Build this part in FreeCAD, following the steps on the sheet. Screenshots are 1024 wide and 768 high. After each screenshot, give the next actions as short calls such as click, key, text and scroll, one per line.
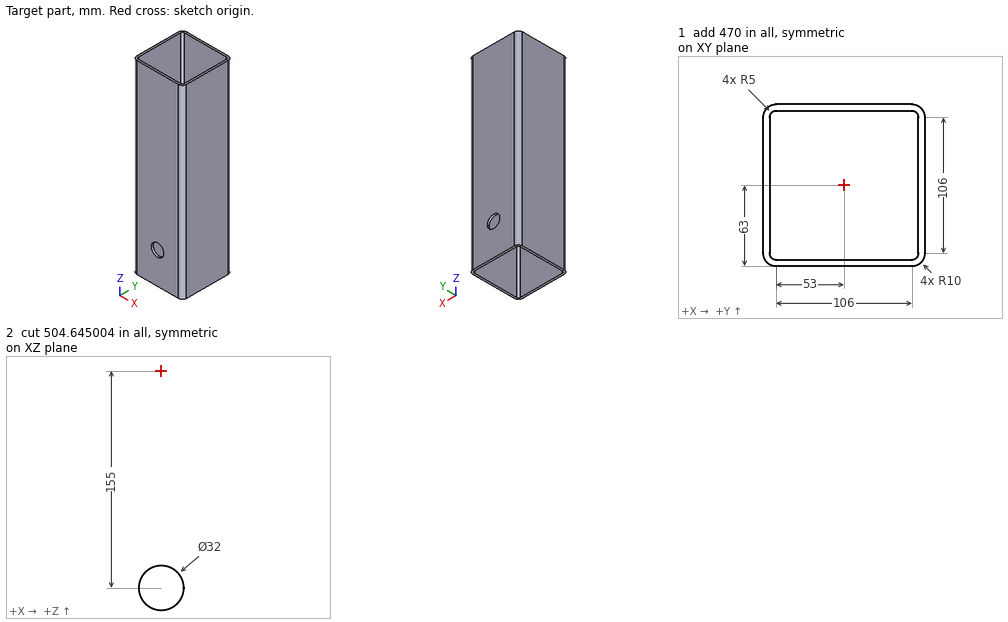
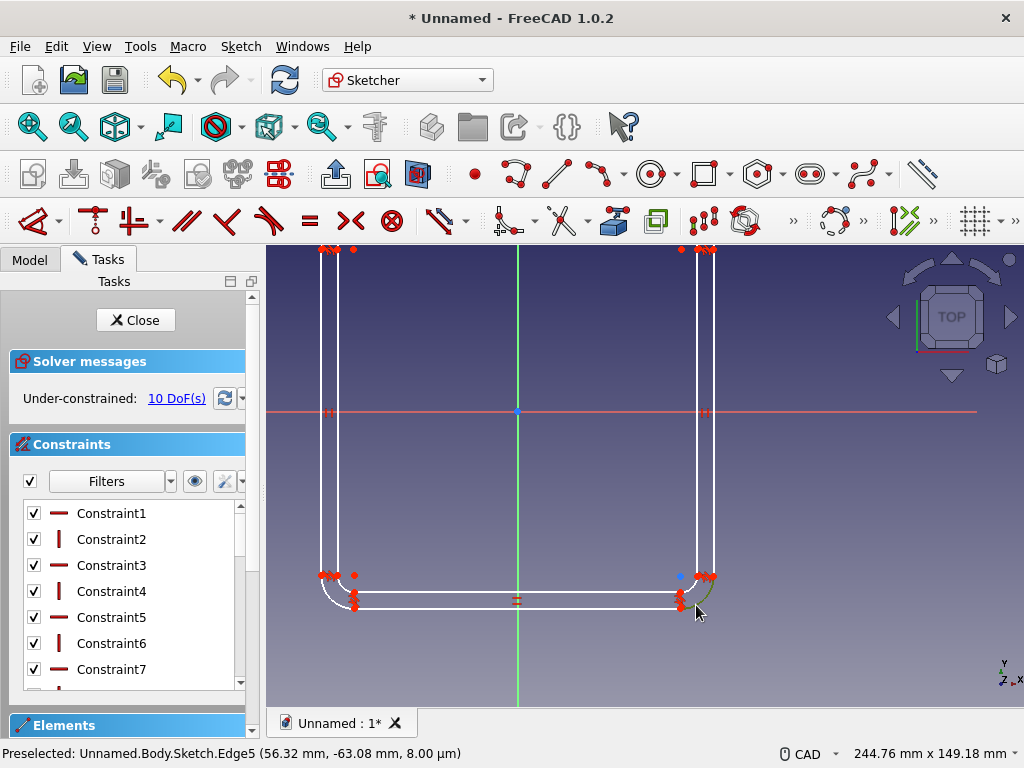
scroll(696, 607, down, 2)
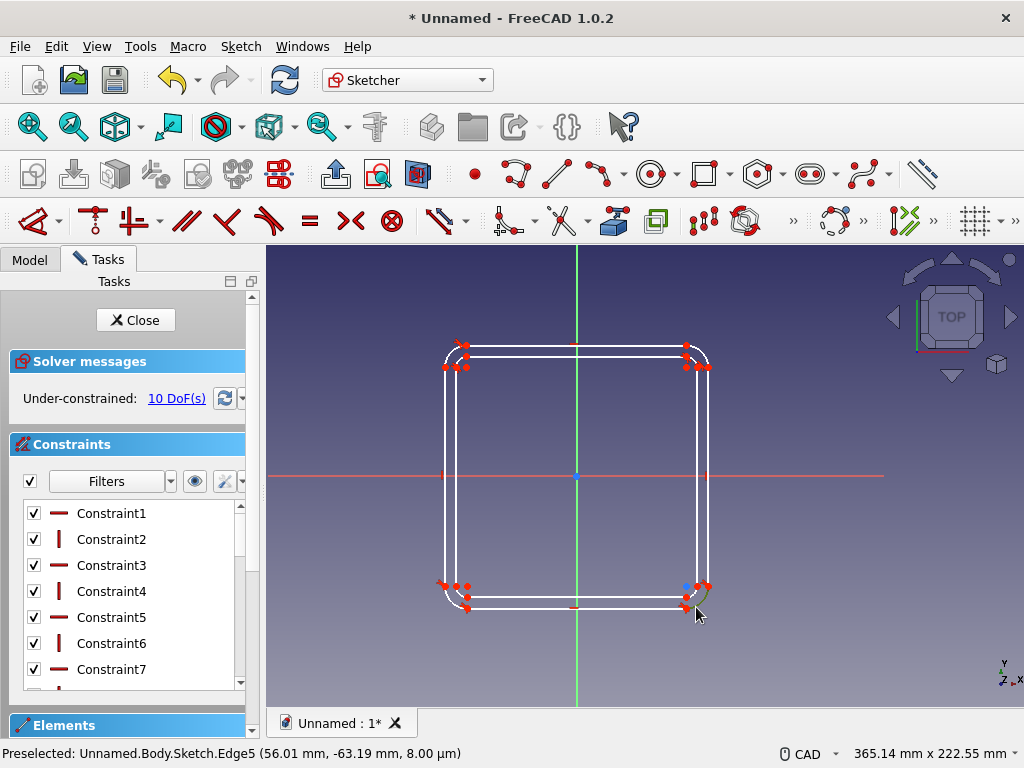
scroll(706, 358, up, 2)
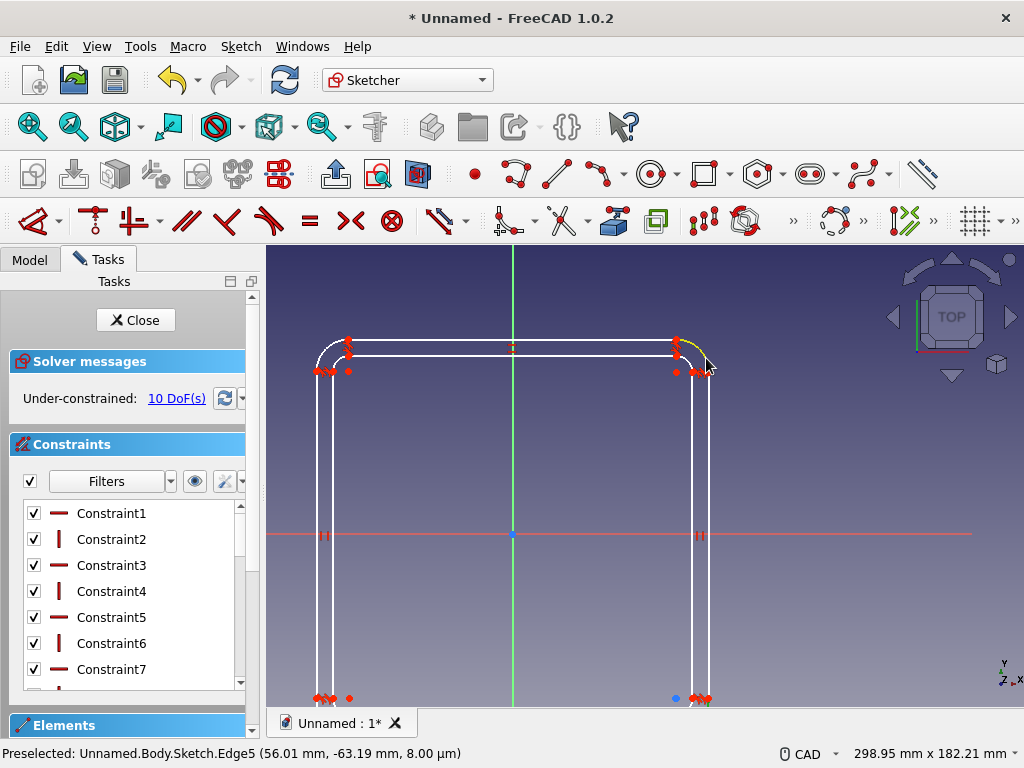
click(705, 357)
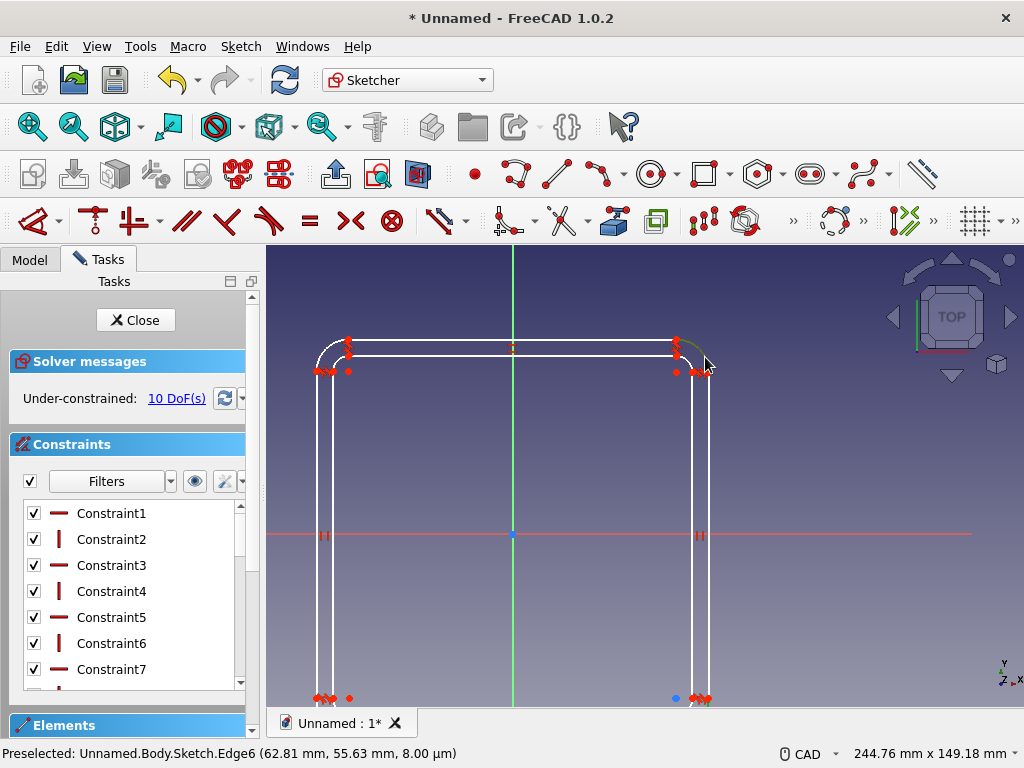
click(334, 343)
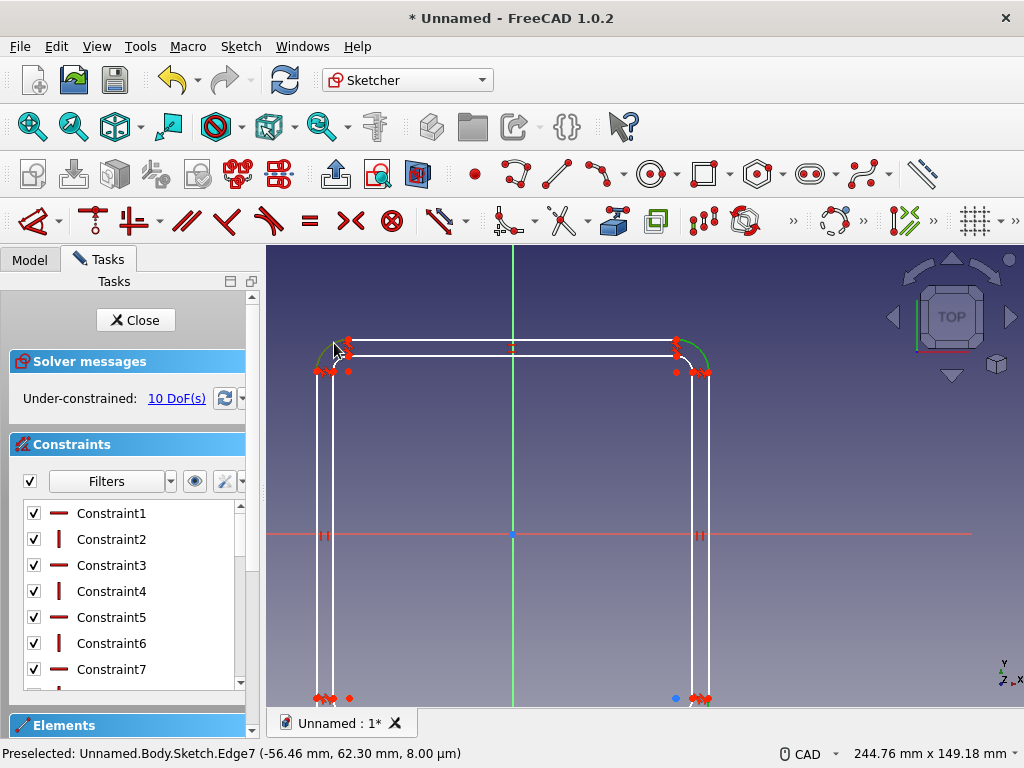
scroll(706, 357, down, 2)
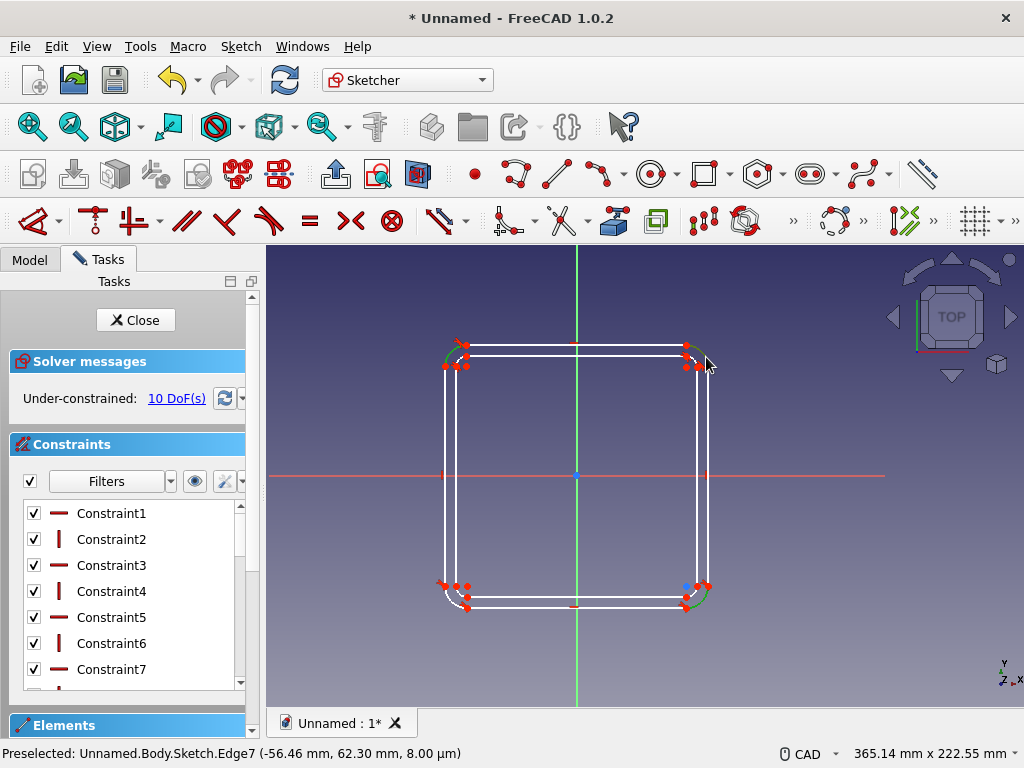
scroll(448, 596, up, 2)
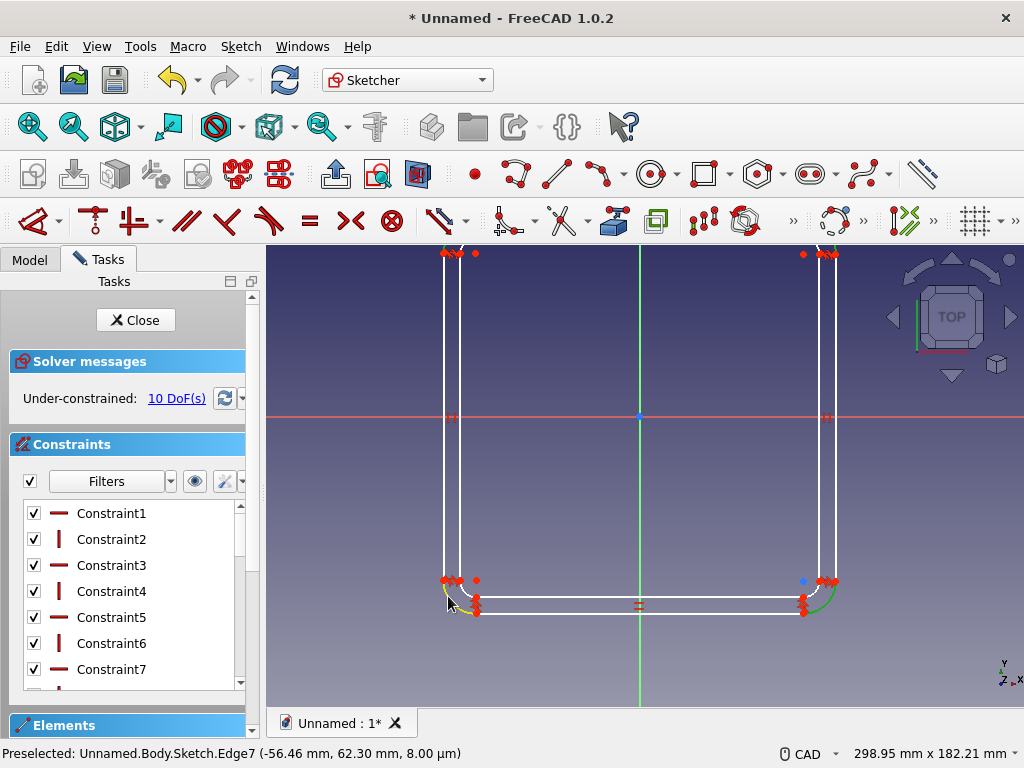
click(447, 596)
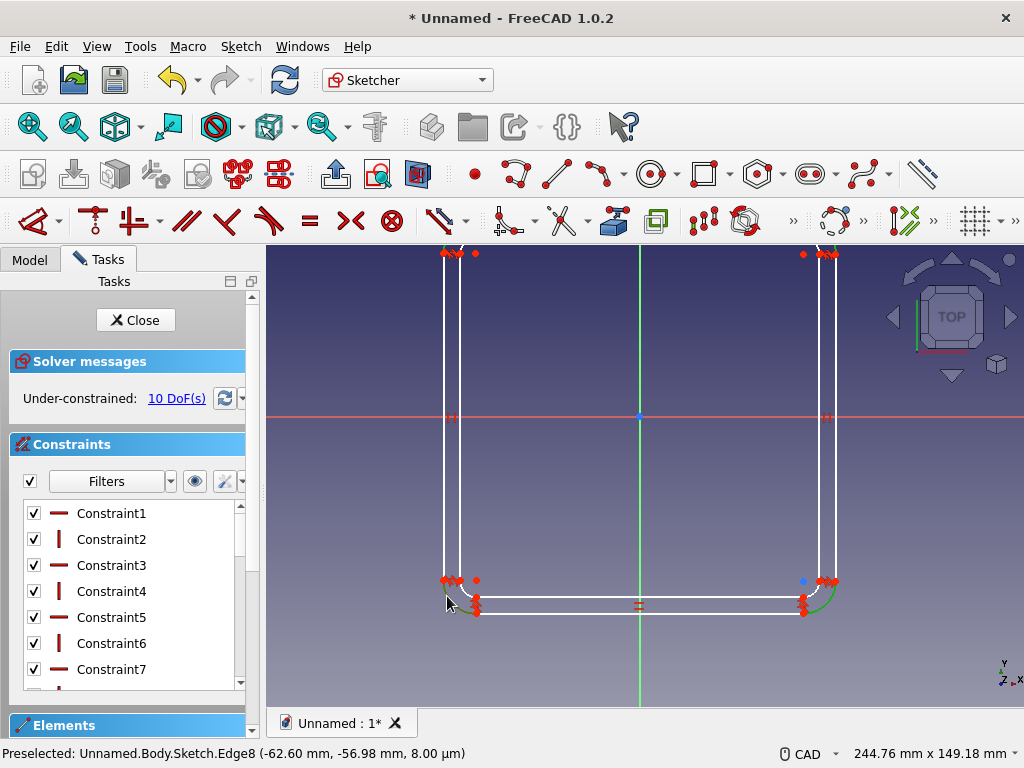
key(e)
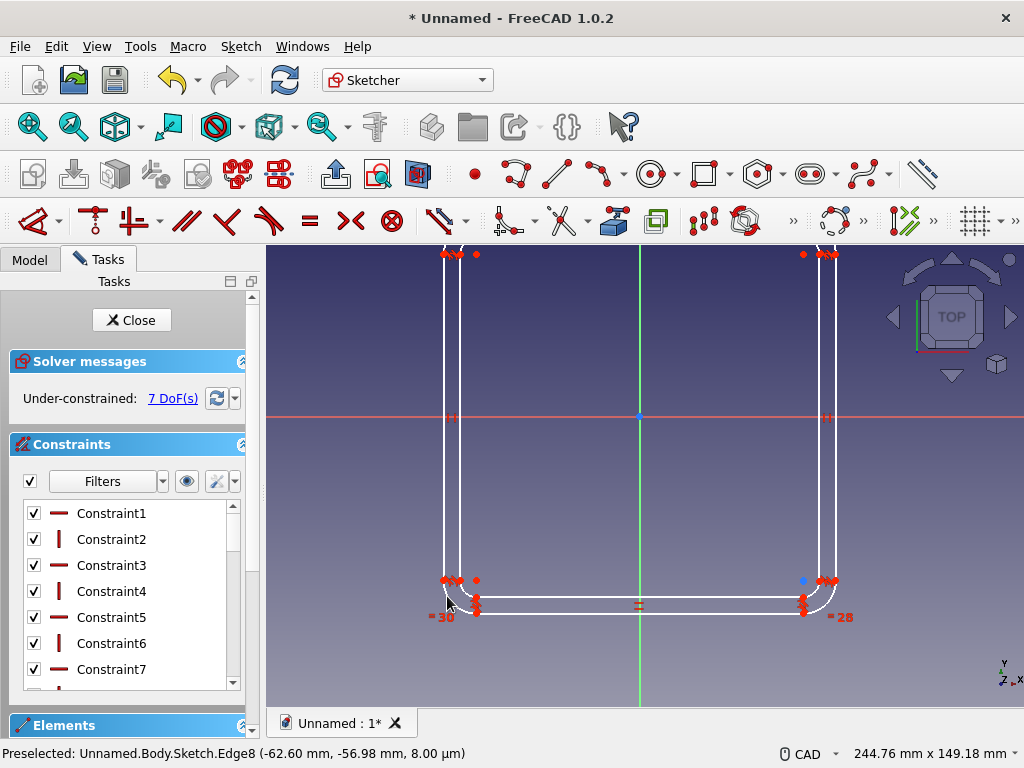
click(465, 592)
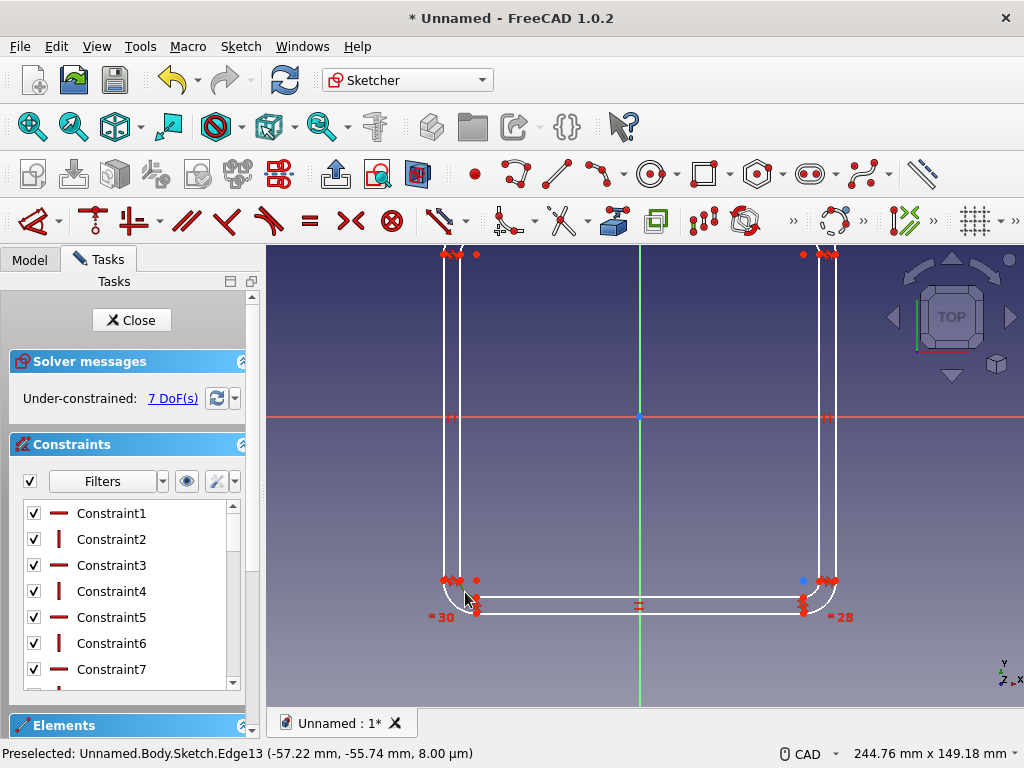
click(815, 592)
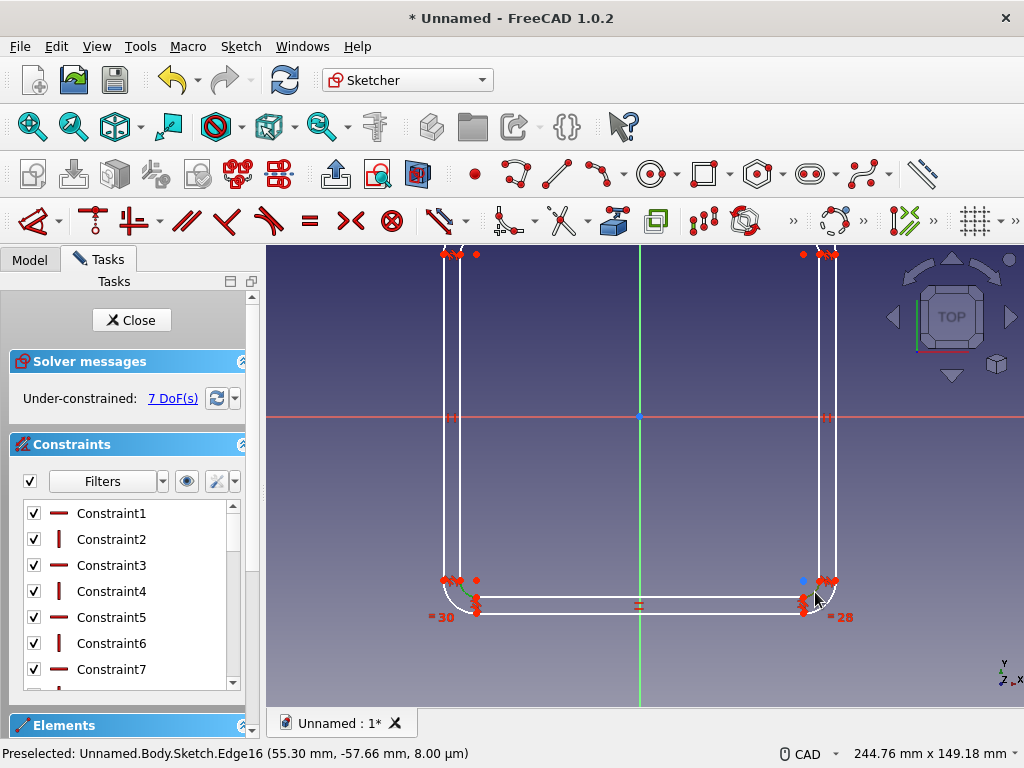
click(310, 222)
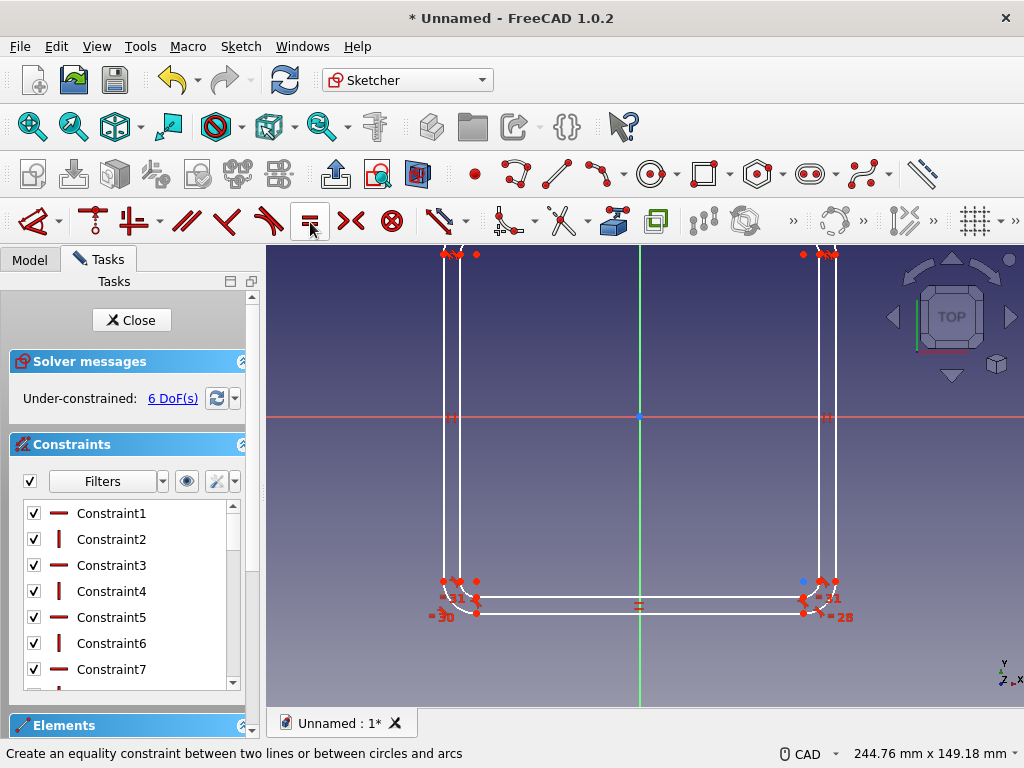
click(32, 222)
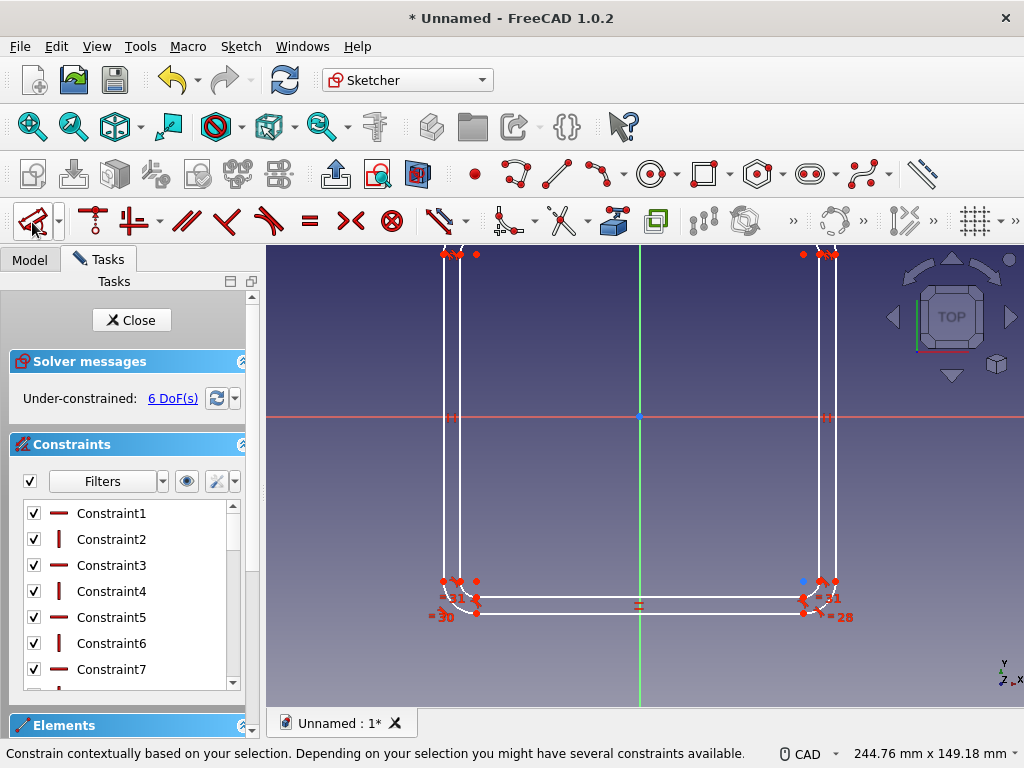
scroll(818, 610, up, 2)